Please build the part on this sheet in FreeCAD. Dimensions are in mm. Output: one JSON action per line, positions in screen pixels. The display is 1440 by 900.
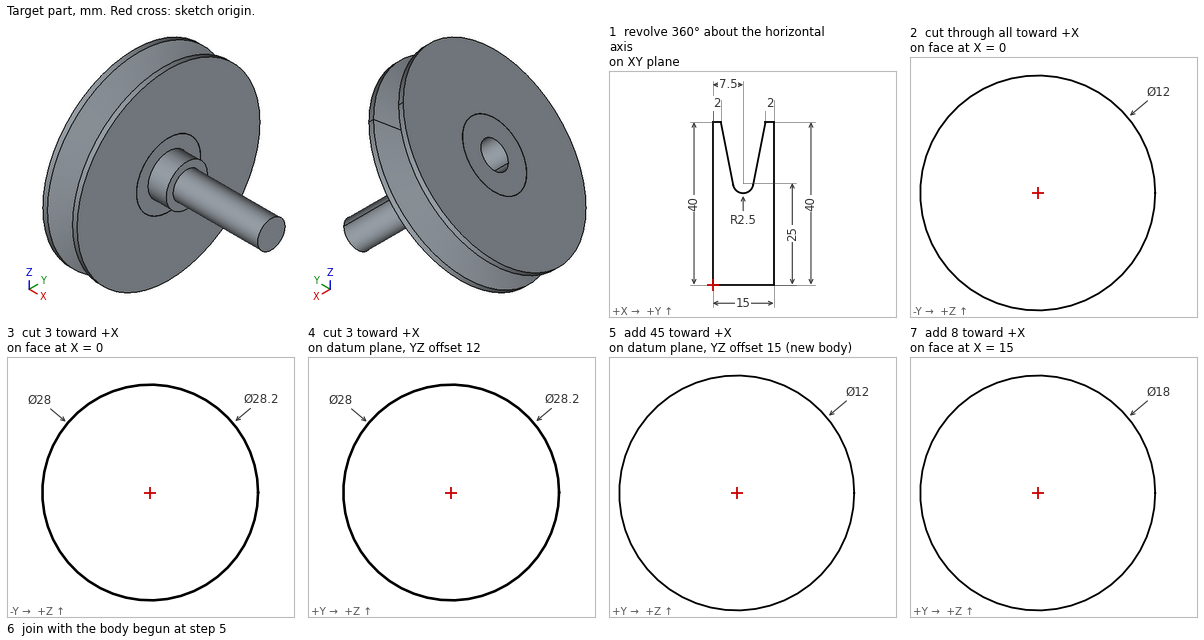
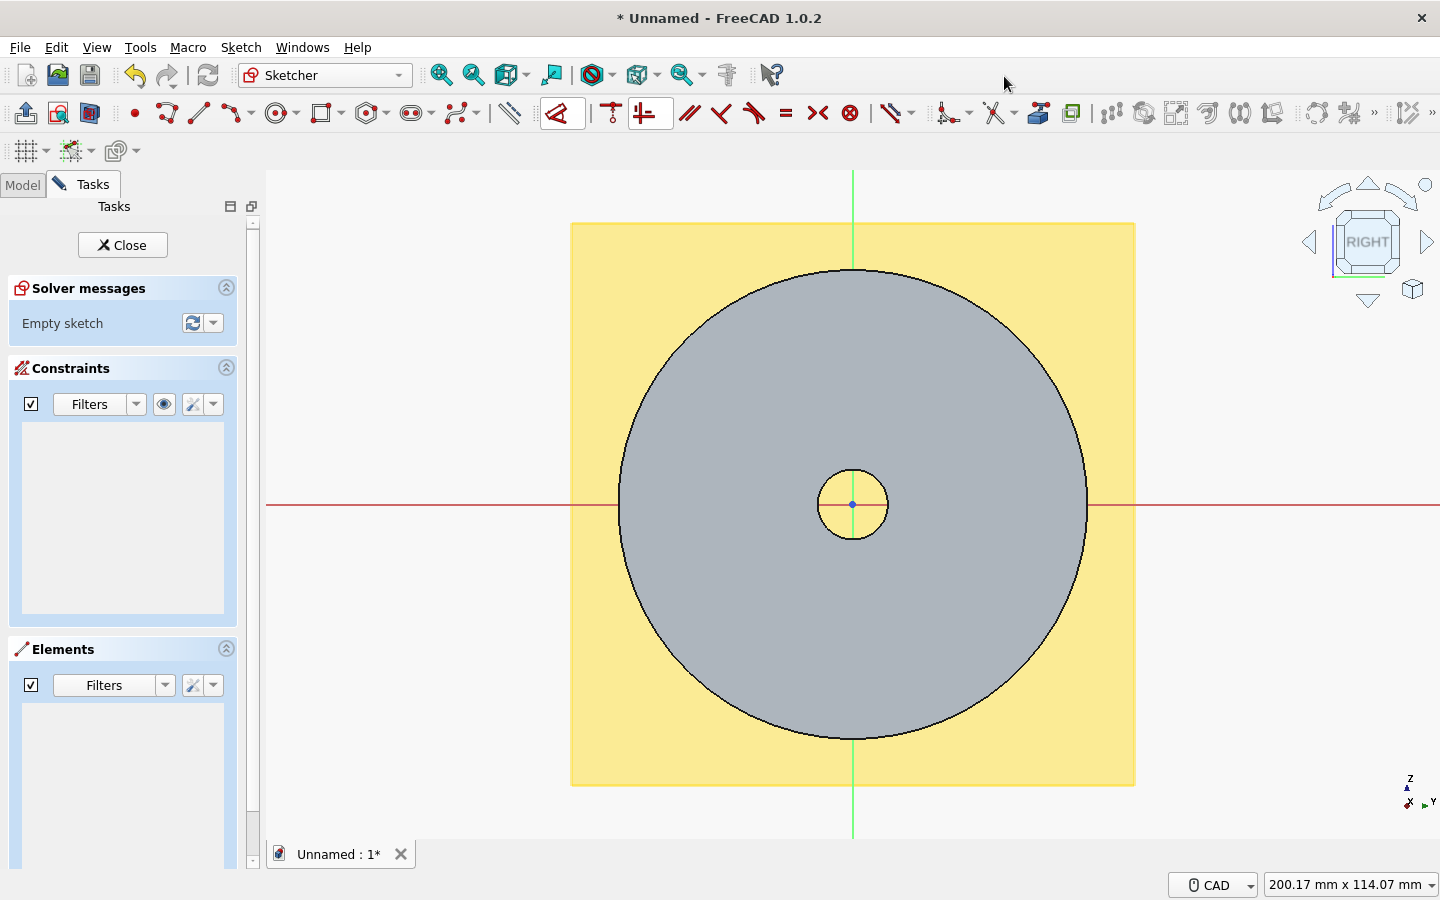
{"action": "left_click", "coordinate": [90, 114]}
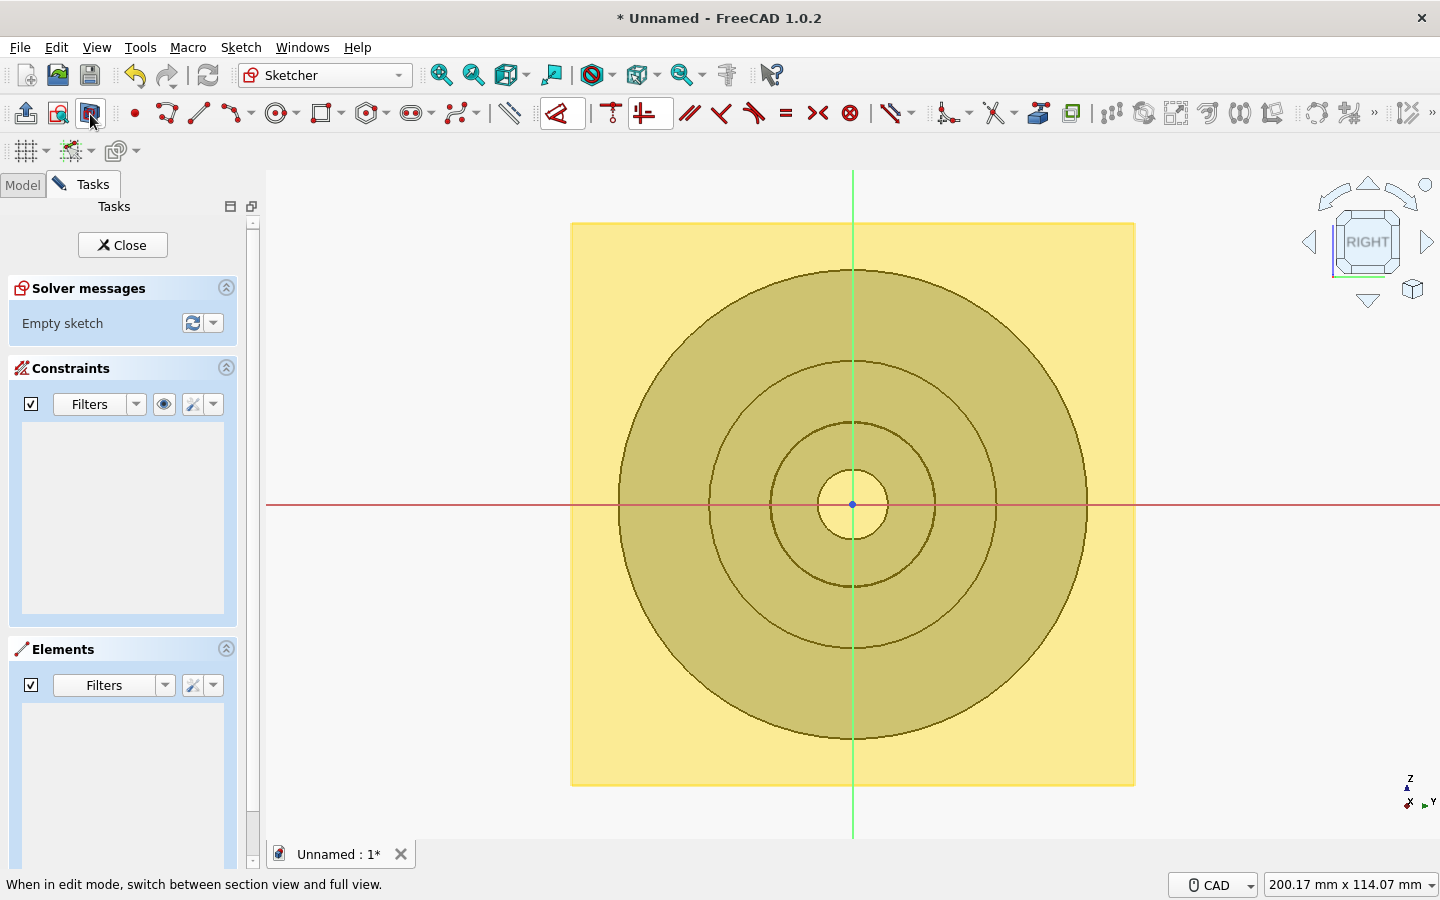
{"action": "scroll", "coordinate": [893, 505], "scroll_direction": "up", "scroll_amount": 5}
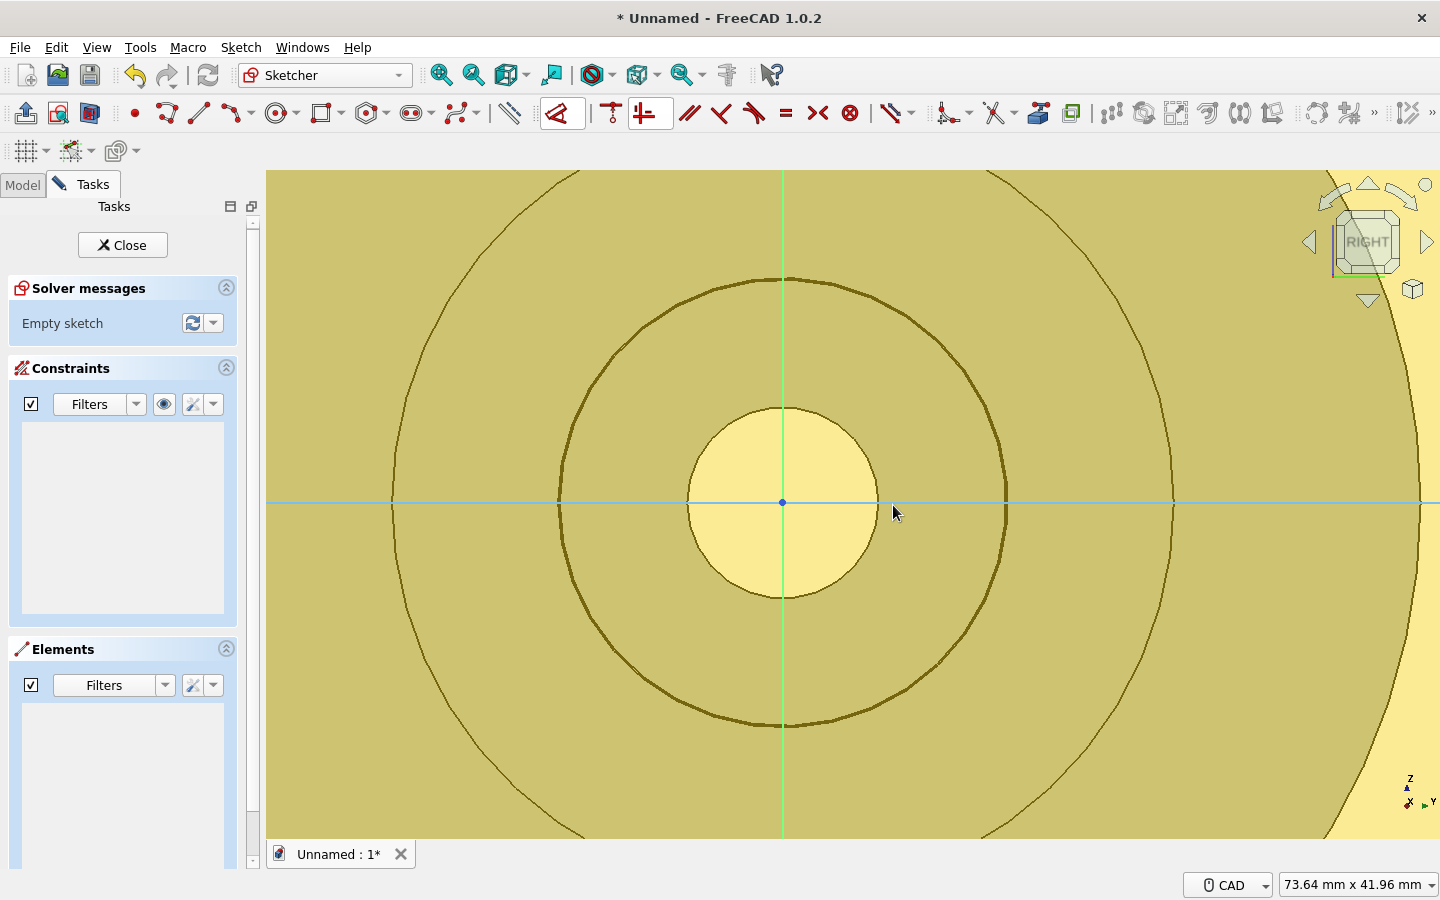
{"action": "key", "text": "g c"}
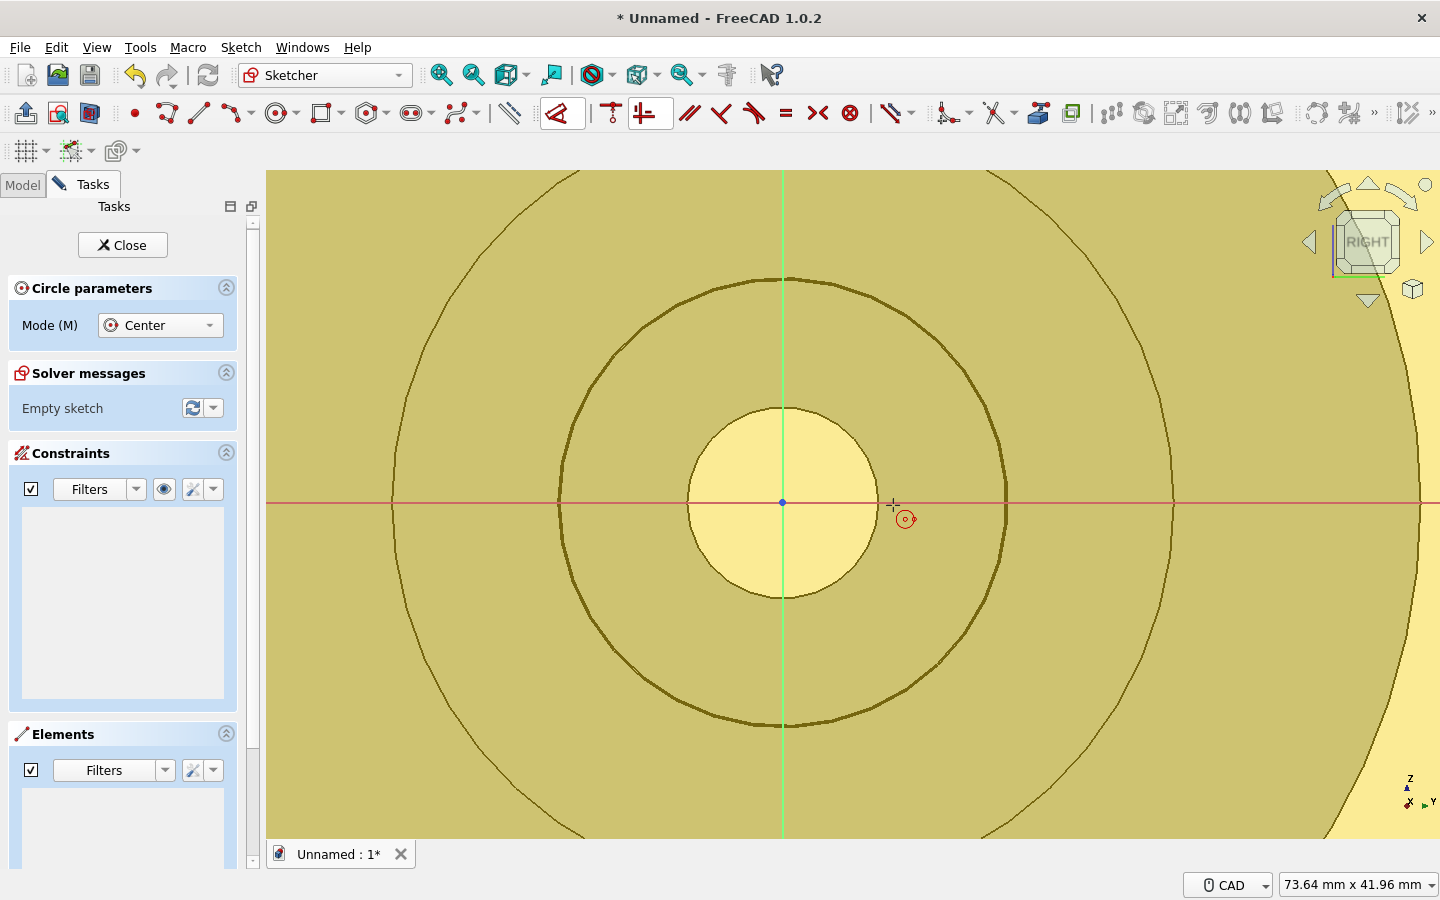
{"action": "left_click", "coordinate": [783, 503]}
{"action": "mouse_move", "coordinate": [942, 344]}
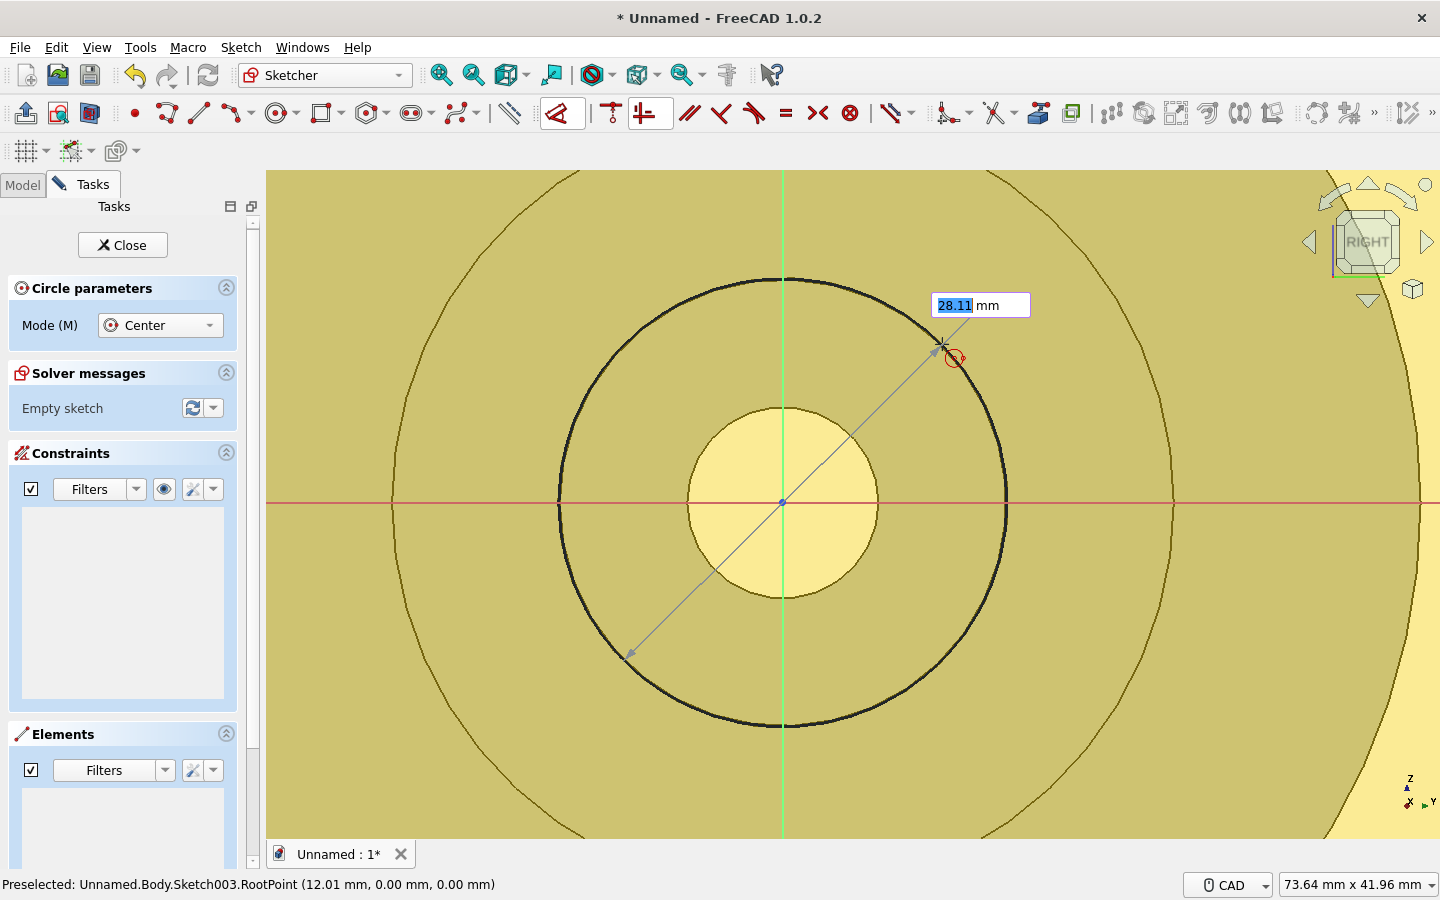
{"action": "type", "text": "28.2"}
{"action": "key", "text": "Return"}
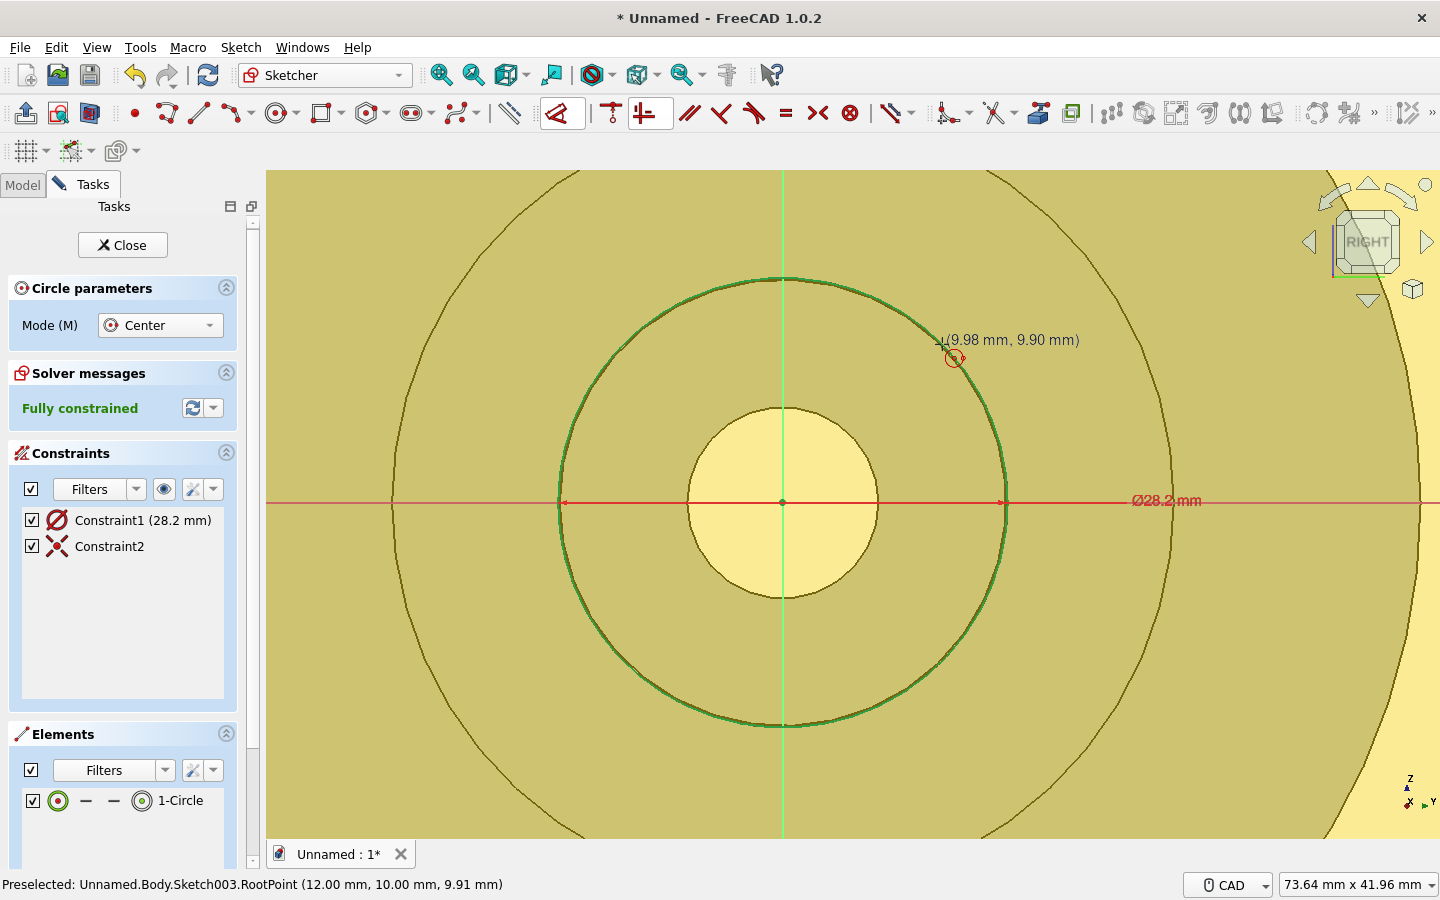
{"action": "left_click", "coordinate": [783, 503]}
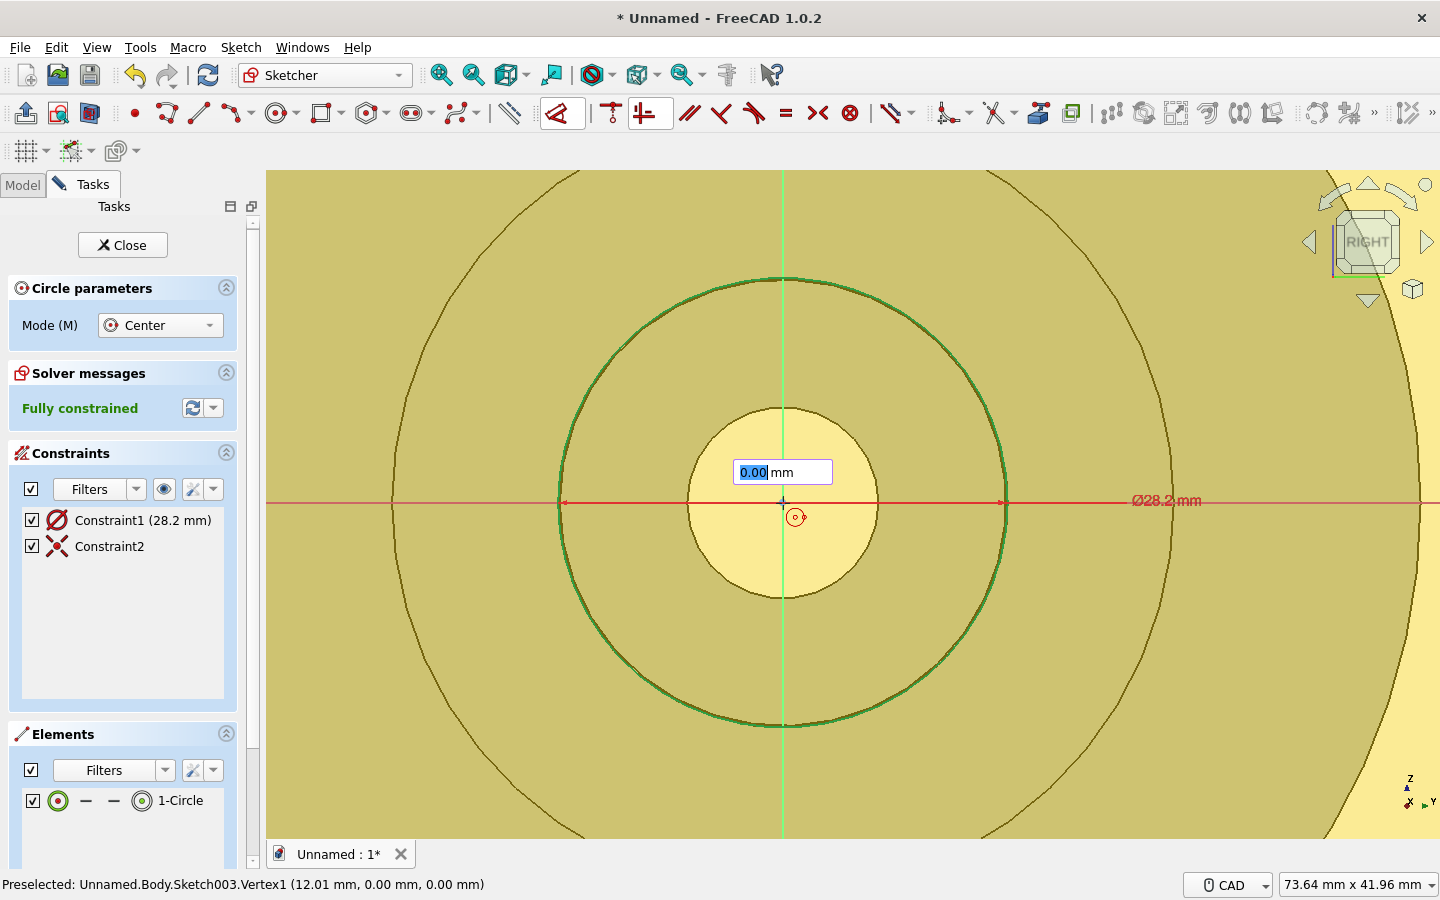
{"action": "scroll", "coordinate": [941, 345], "scroll_direction": "up", "scroll_amount": 12}
{"action": "mouse_move", "coordinate": [932, 342]}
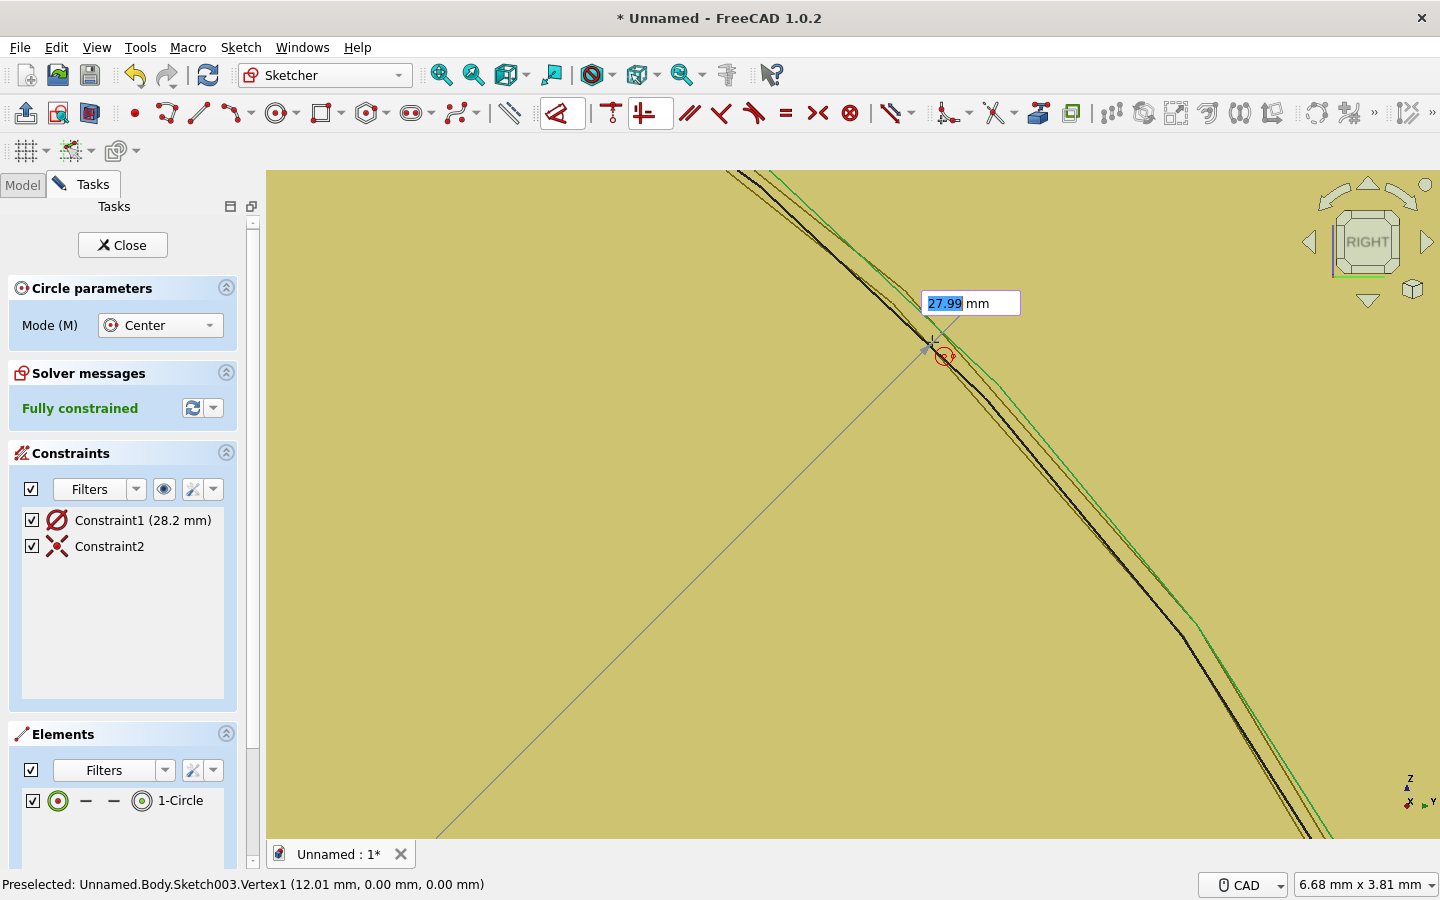
{"action": "type", "text": "28"}
{"action": "key", "text": "Return"}
{"action": "key", "text": "Escape"}